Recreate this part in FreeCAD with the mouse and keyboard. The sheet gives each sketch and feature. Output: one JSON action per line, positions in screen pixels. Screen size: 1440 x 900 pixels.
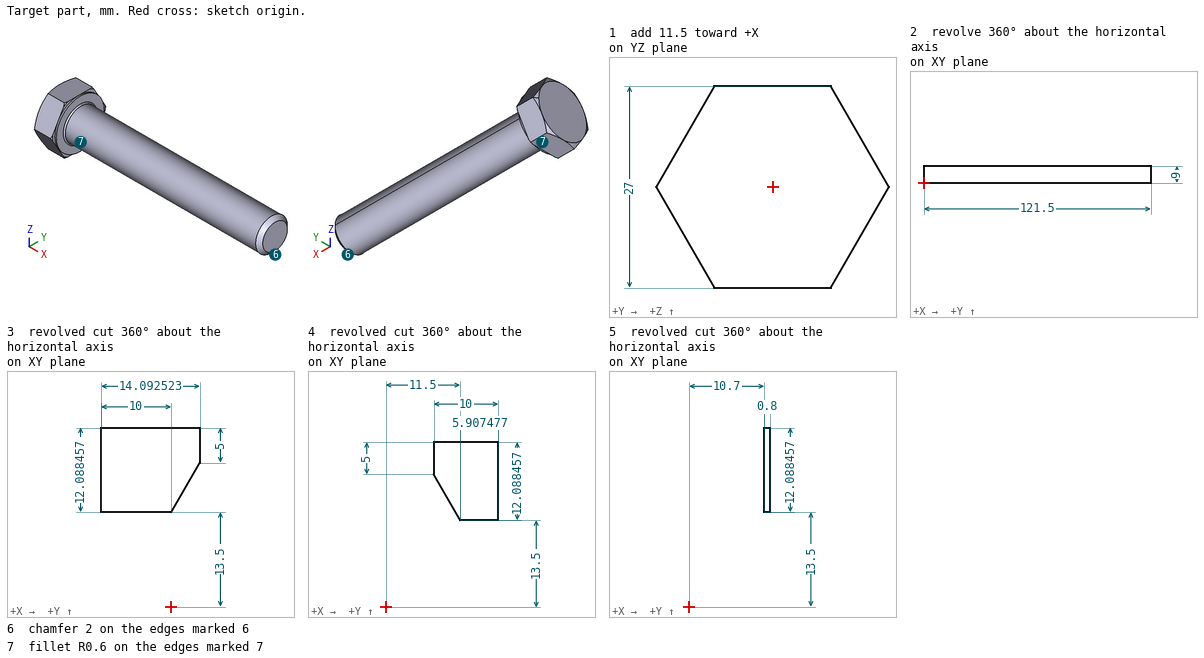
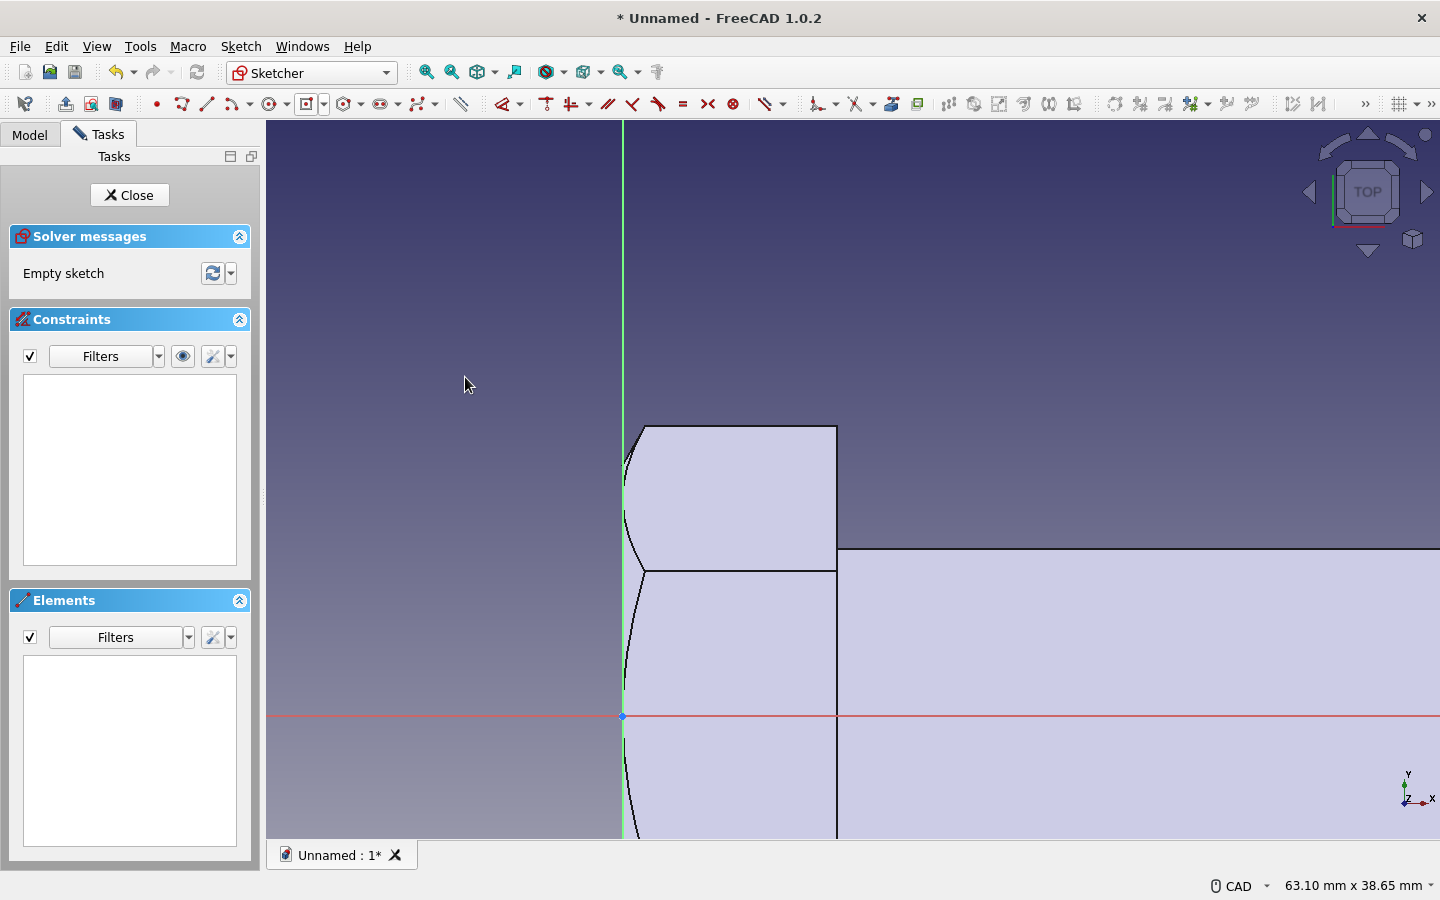
{"action": "left_click", "coordinate": [182, 104]}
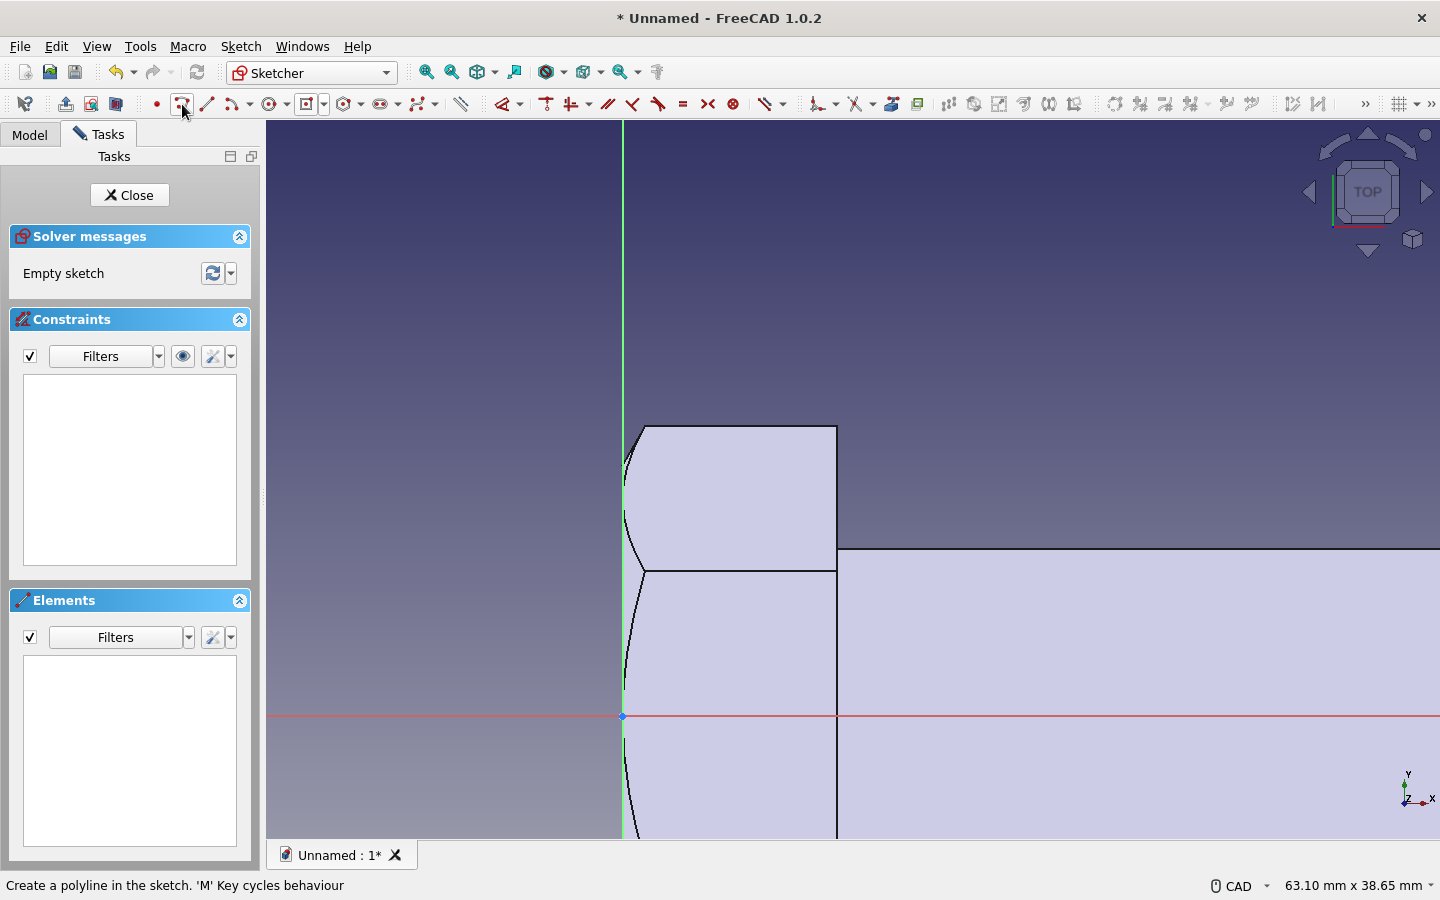
{"action": "left_click", "coordinate": [837, 465]}
{"action": "left_click", "coordinate": [946, 465]}
{"action": "left_click", "coordinate": [946, 240]}
{"action": "left_click", "coordinate": [760, 240]}
{"action": "left_click", "coordinate": [760, 333]}
{"action": "left_click", "coordinate": [837, 466]}
{"action": "key", "text": "Escape"}
{"action": "key", "text": "Escape"}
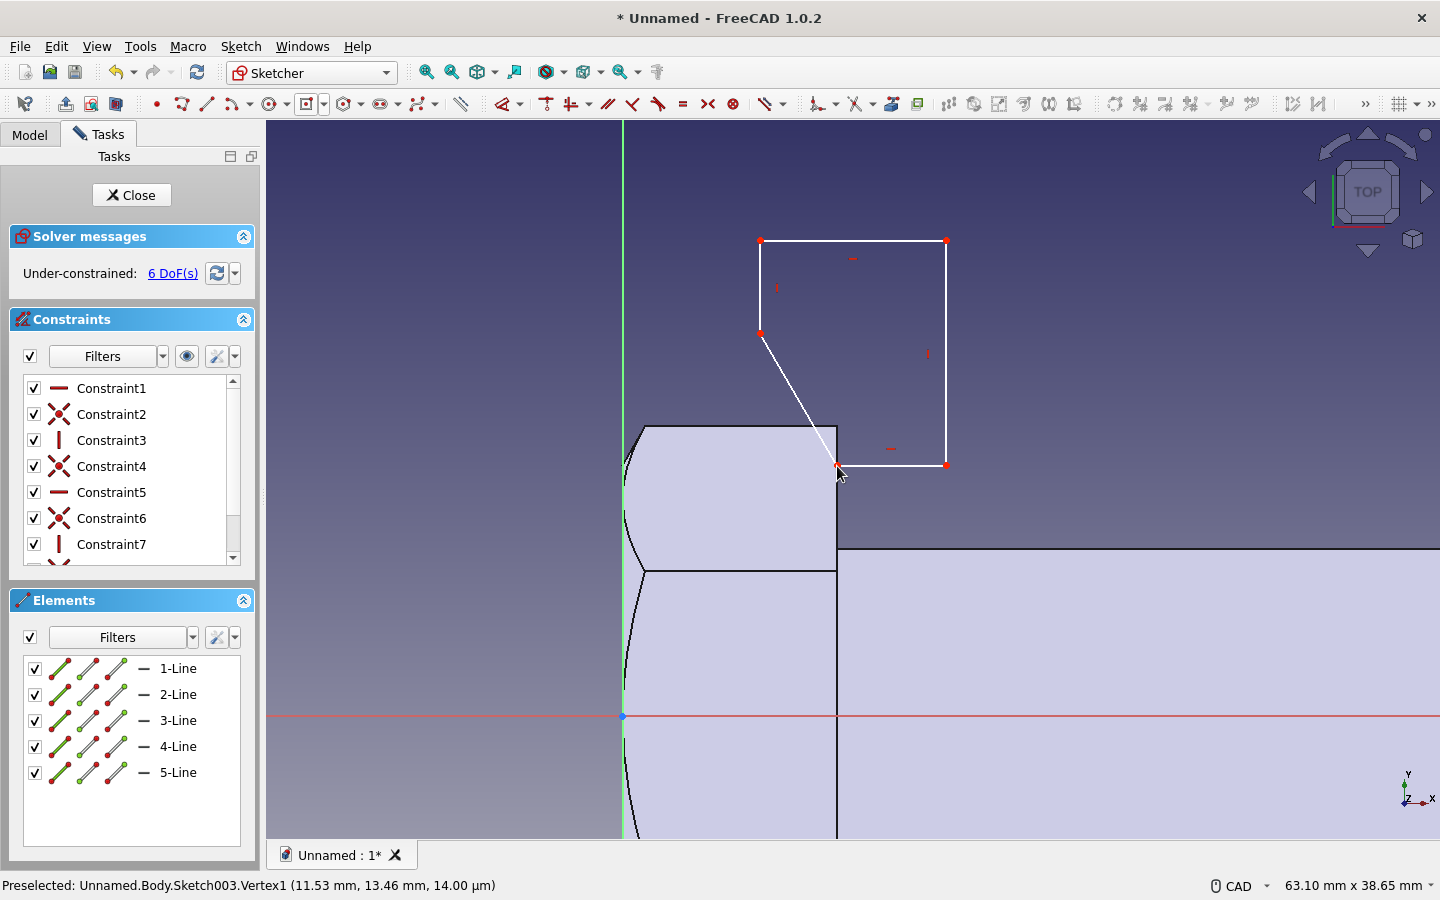
{"action": "left_click", "coordinate": [502, 104]}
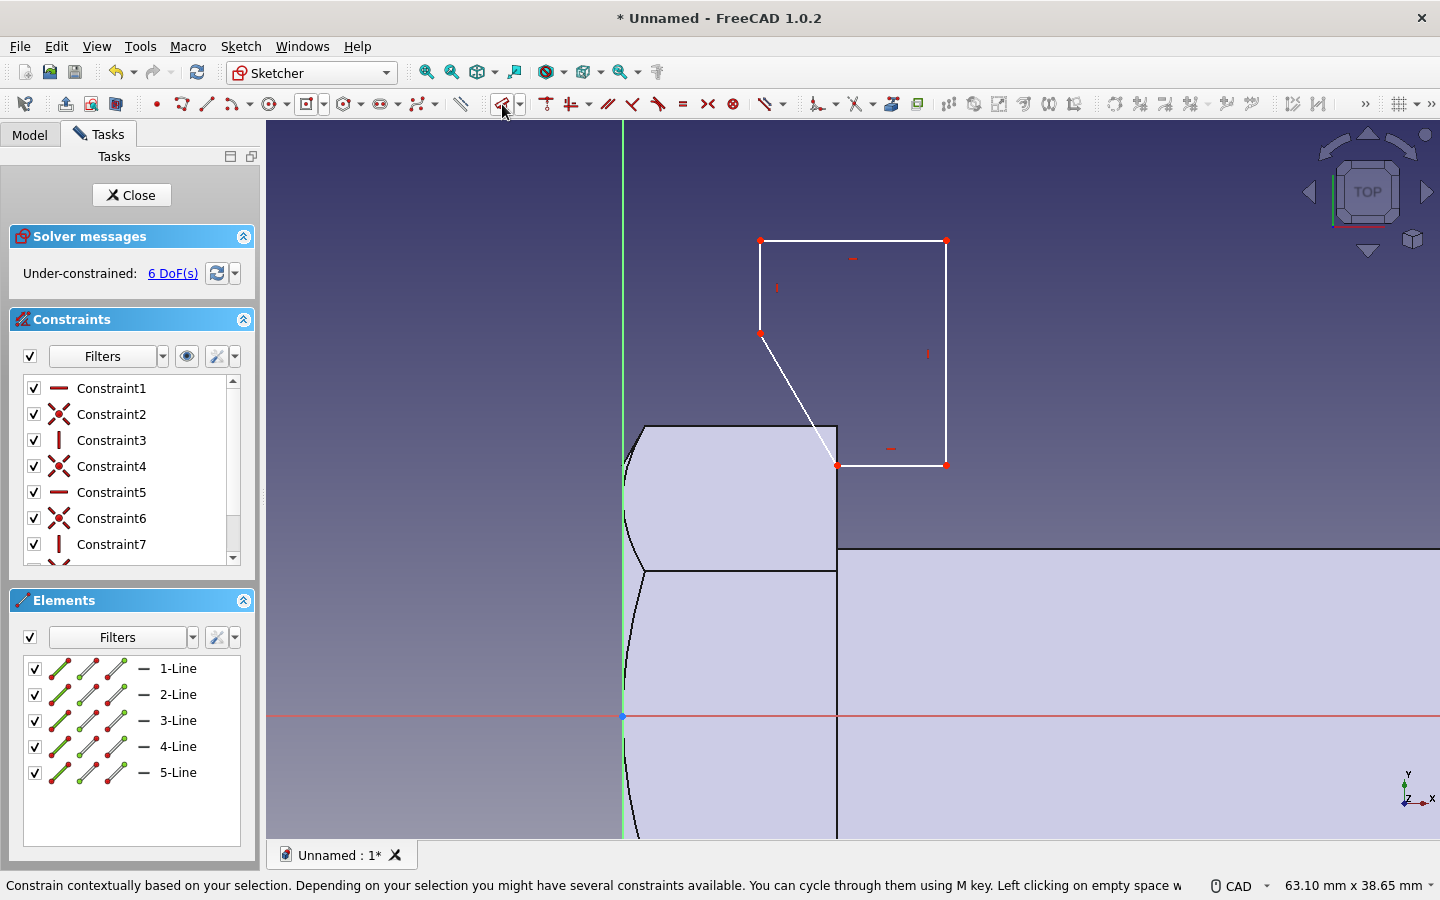
{"action": "left_click", "coordinate": [760, 269]}
{"action": "left_click", "coordinate": [726, 288]}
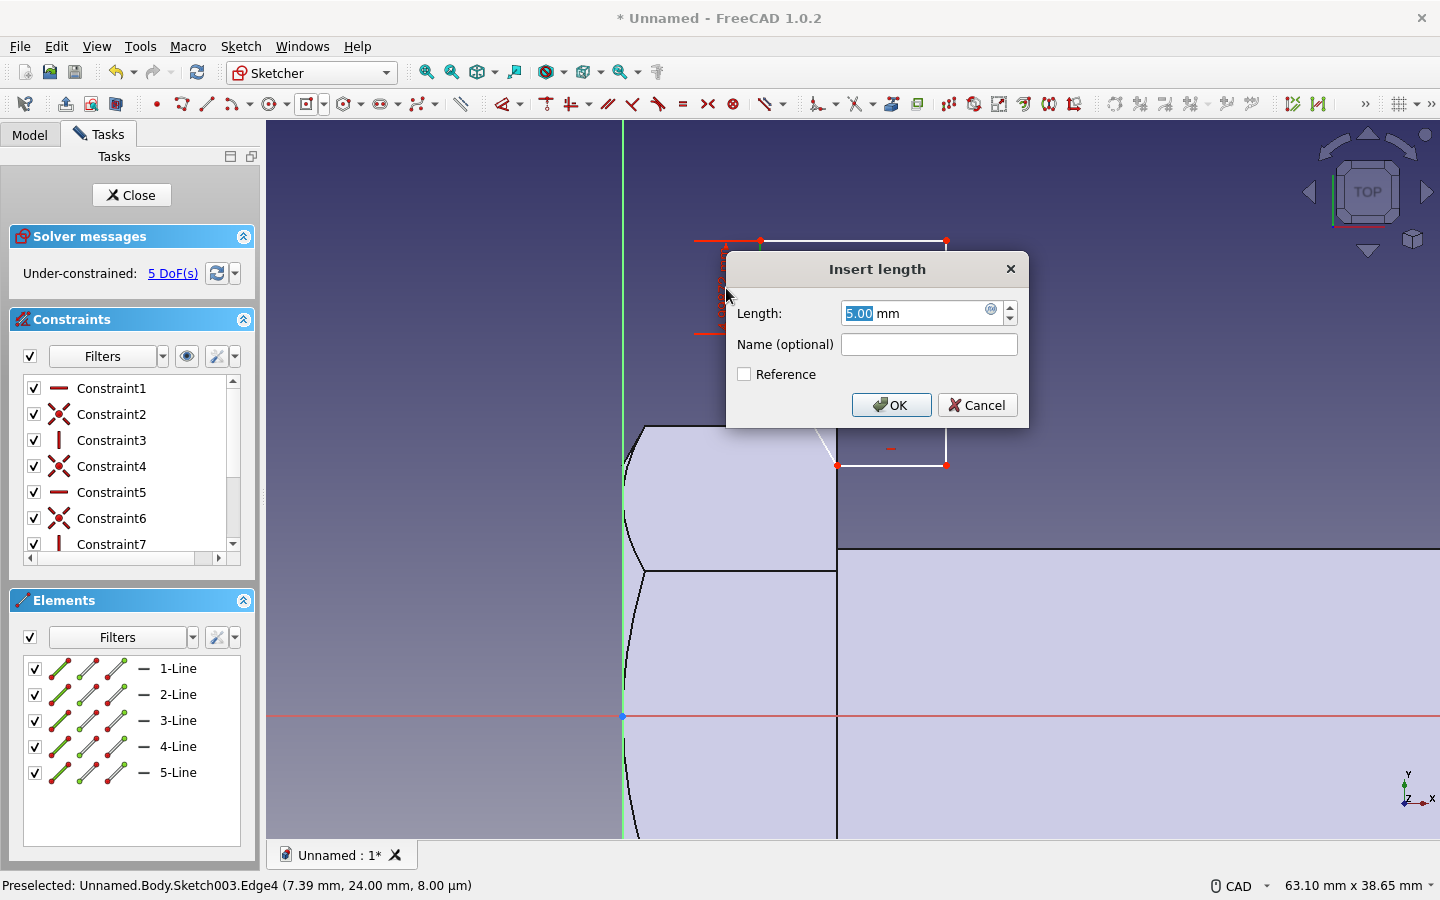
{"action": "type", "text": "5"}
{"action": "key", "text": "Return"}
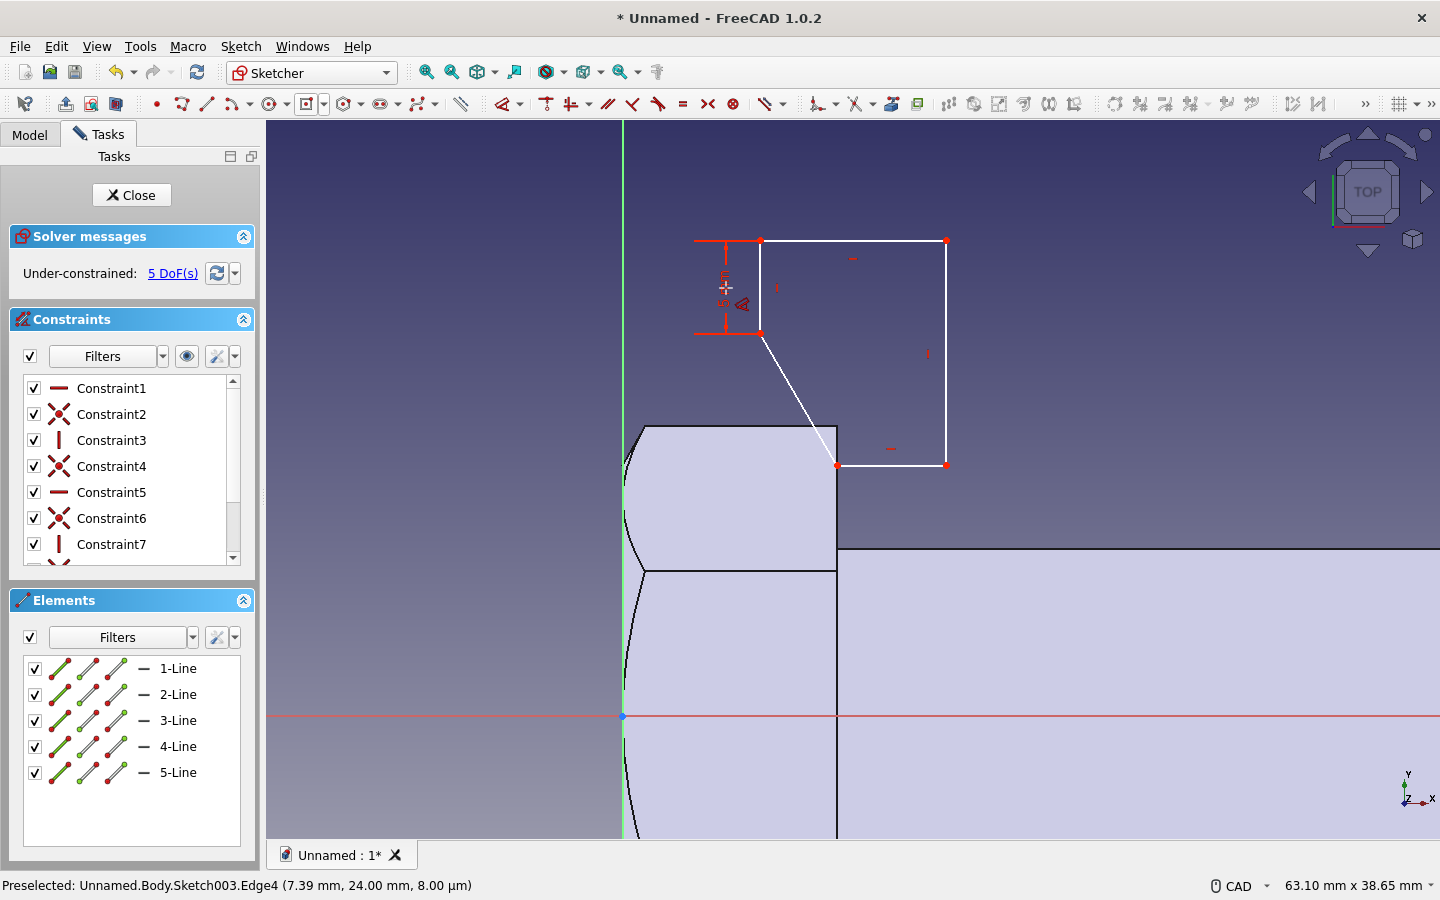
{"action": "left_click", "coordinate": [890, 241]}
{"action": "left_click", "coordinate": [853, 207]}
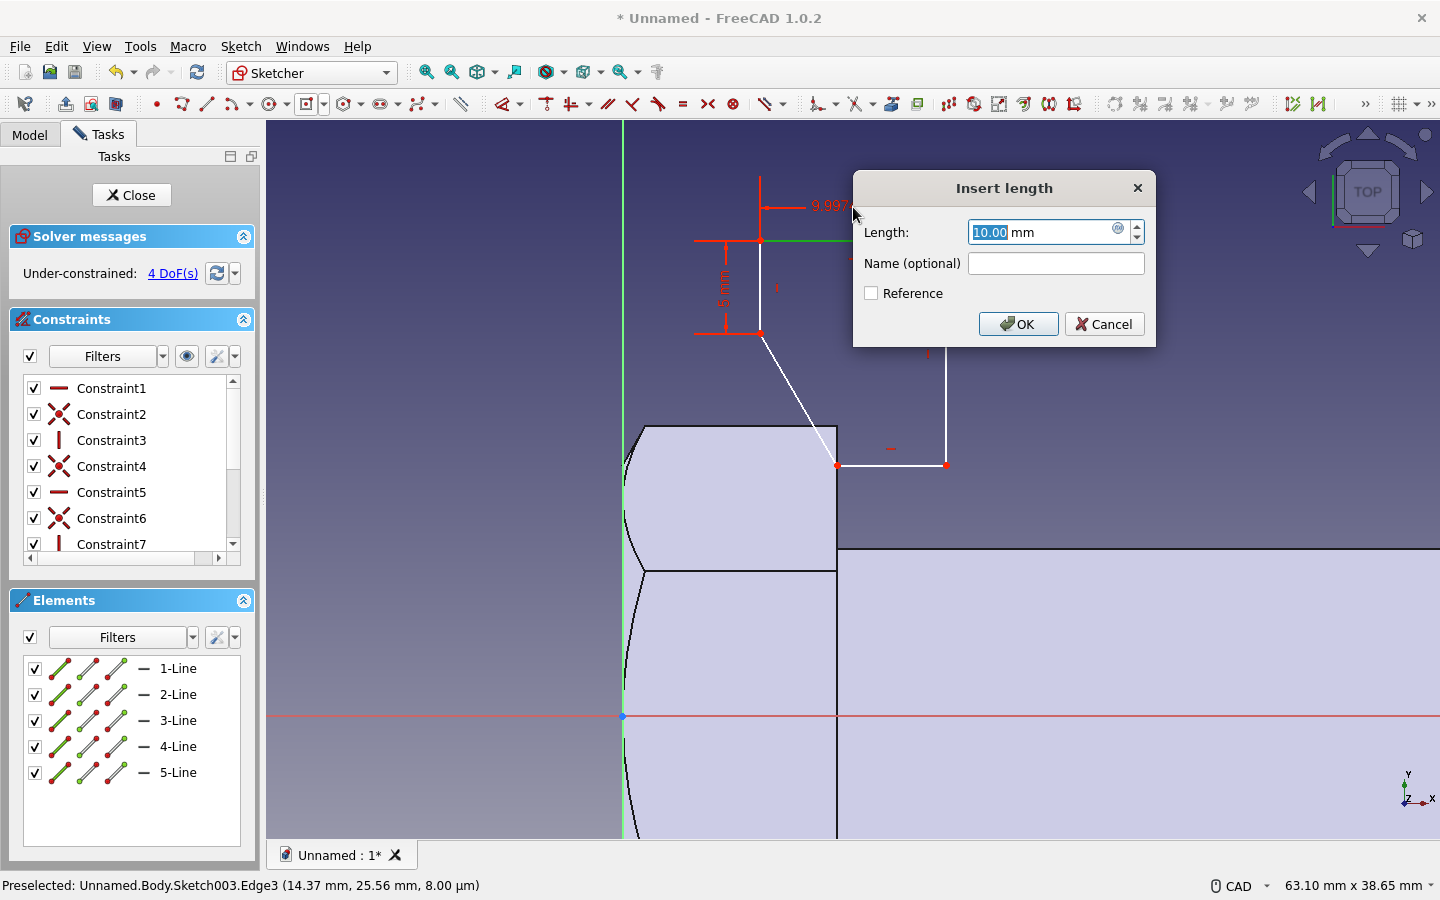
{"action": "type", "text": "10"}
{"action": "key", "text": "Return"}